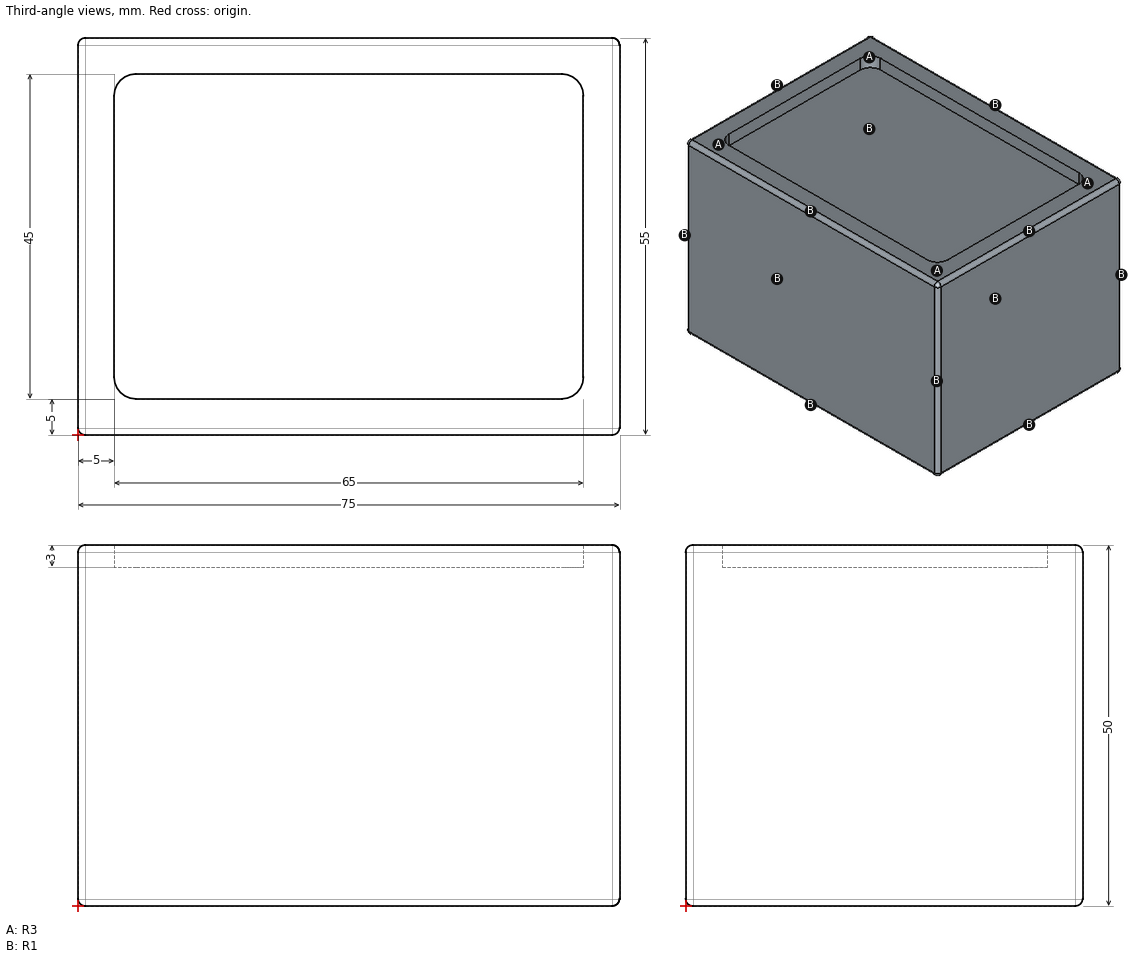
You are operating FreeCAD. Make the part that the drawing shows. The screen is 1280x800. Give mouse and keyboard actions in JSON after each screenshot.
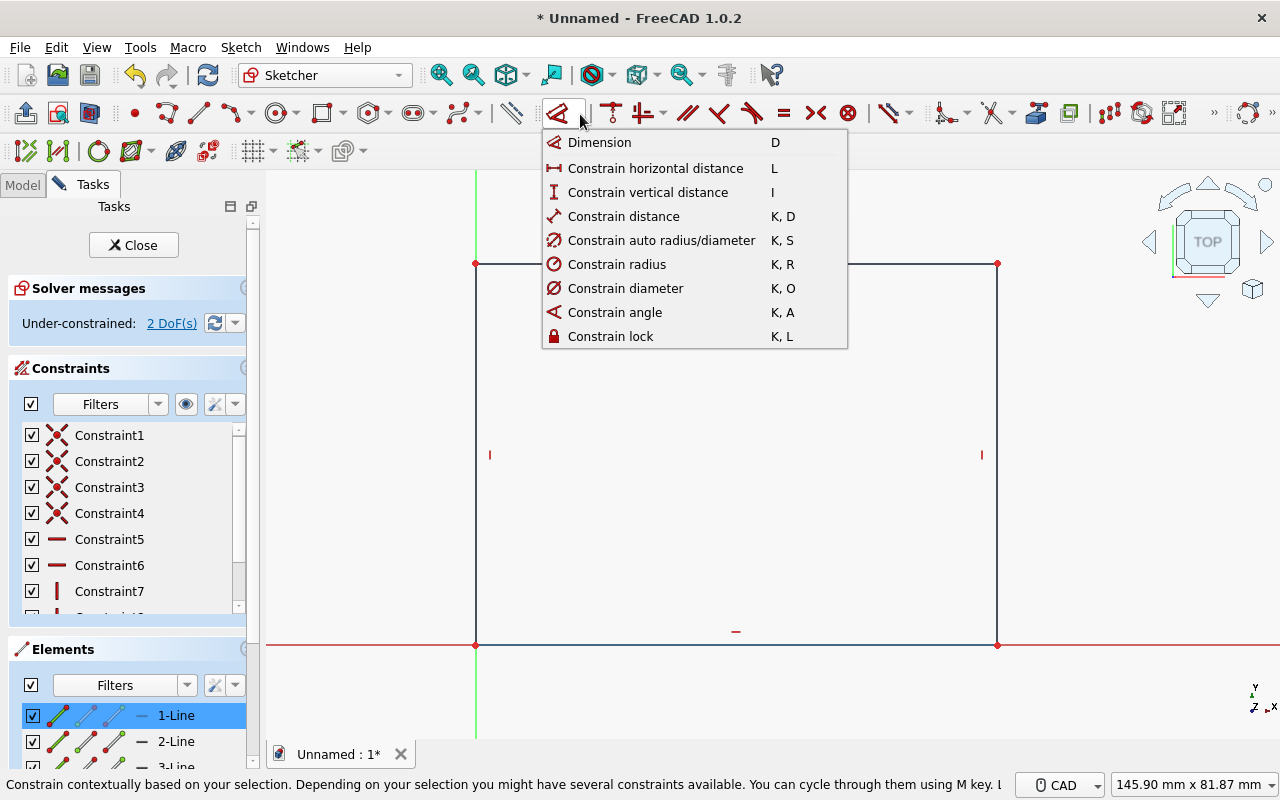
{"action": "left_click", "coordinate": [695, 168]}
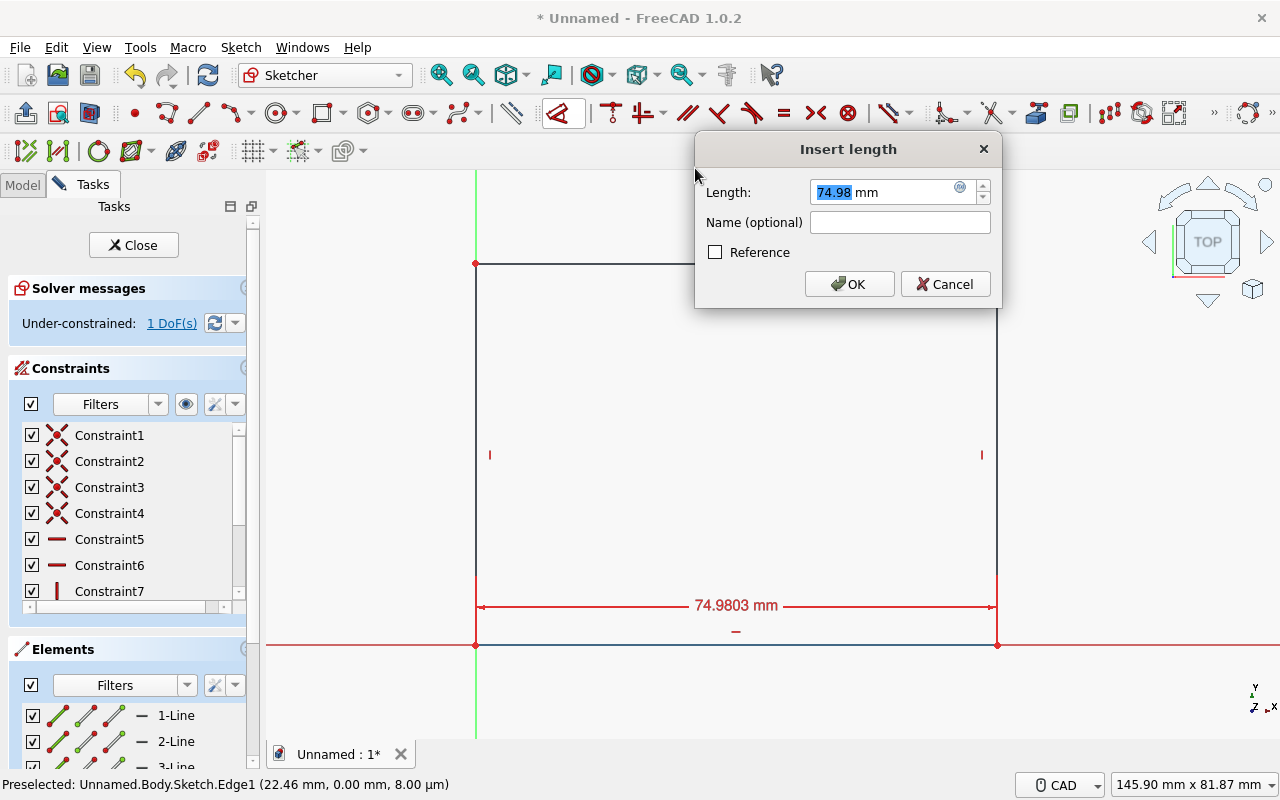
{"action": "type", "text": "75"}
{"action": "key", "text": "Return"}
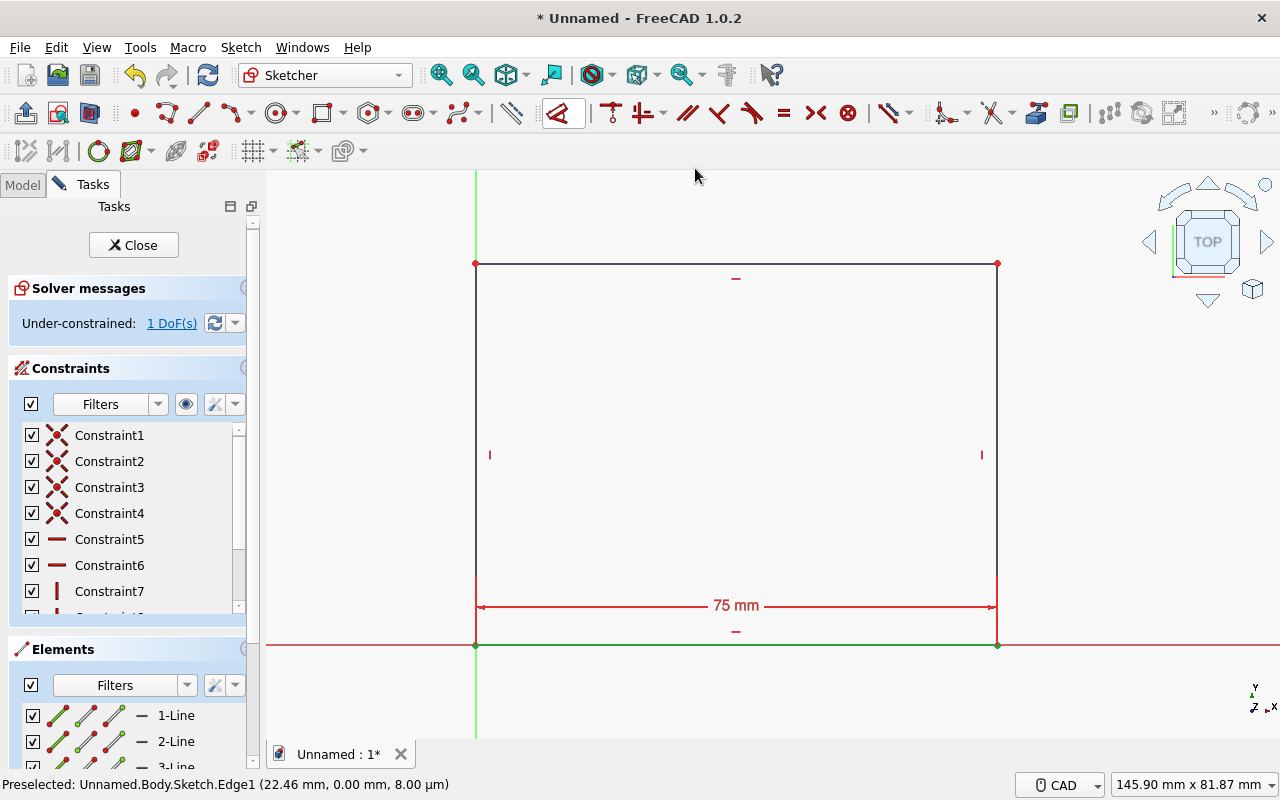
{"action": "left_click", "coordinate": [997, 531]}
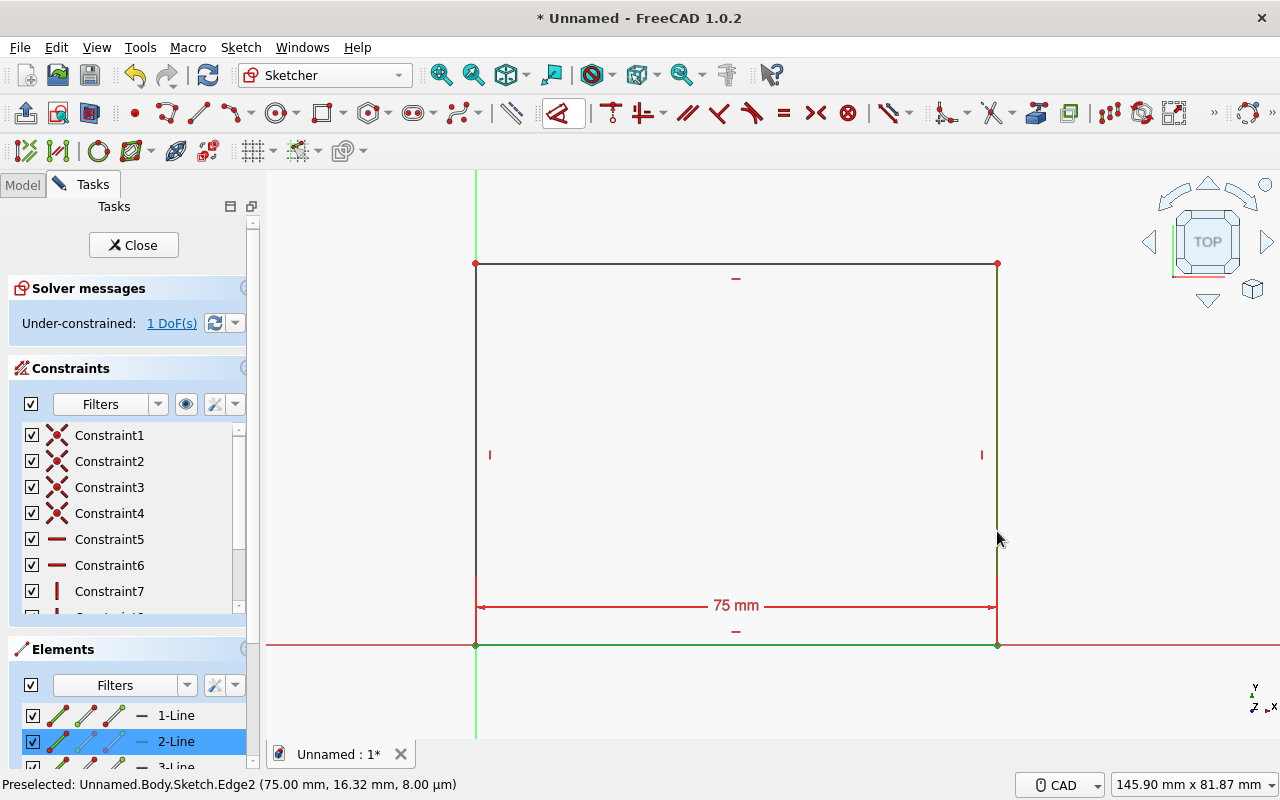
{"action": "left_click", "coordinate": [580, 114]}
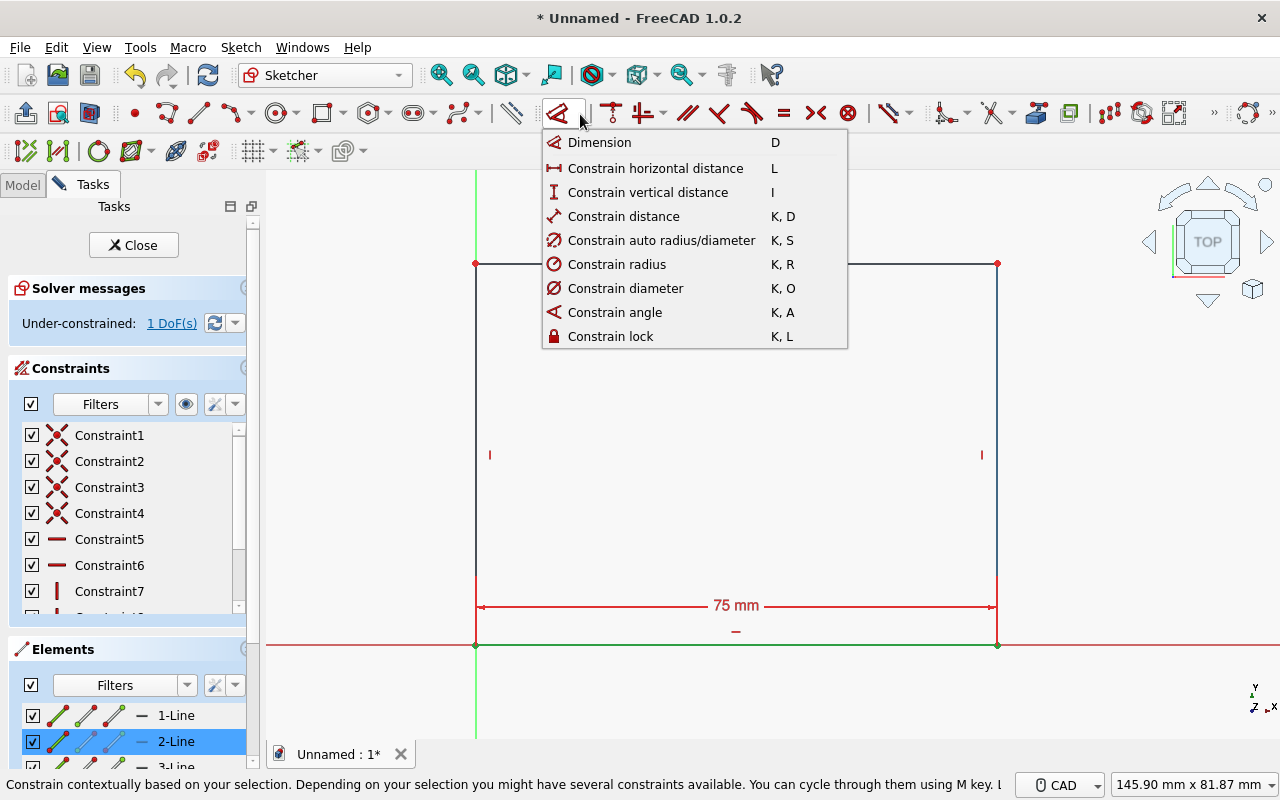
{"action": "left_click", "coordinate": [695, 192]}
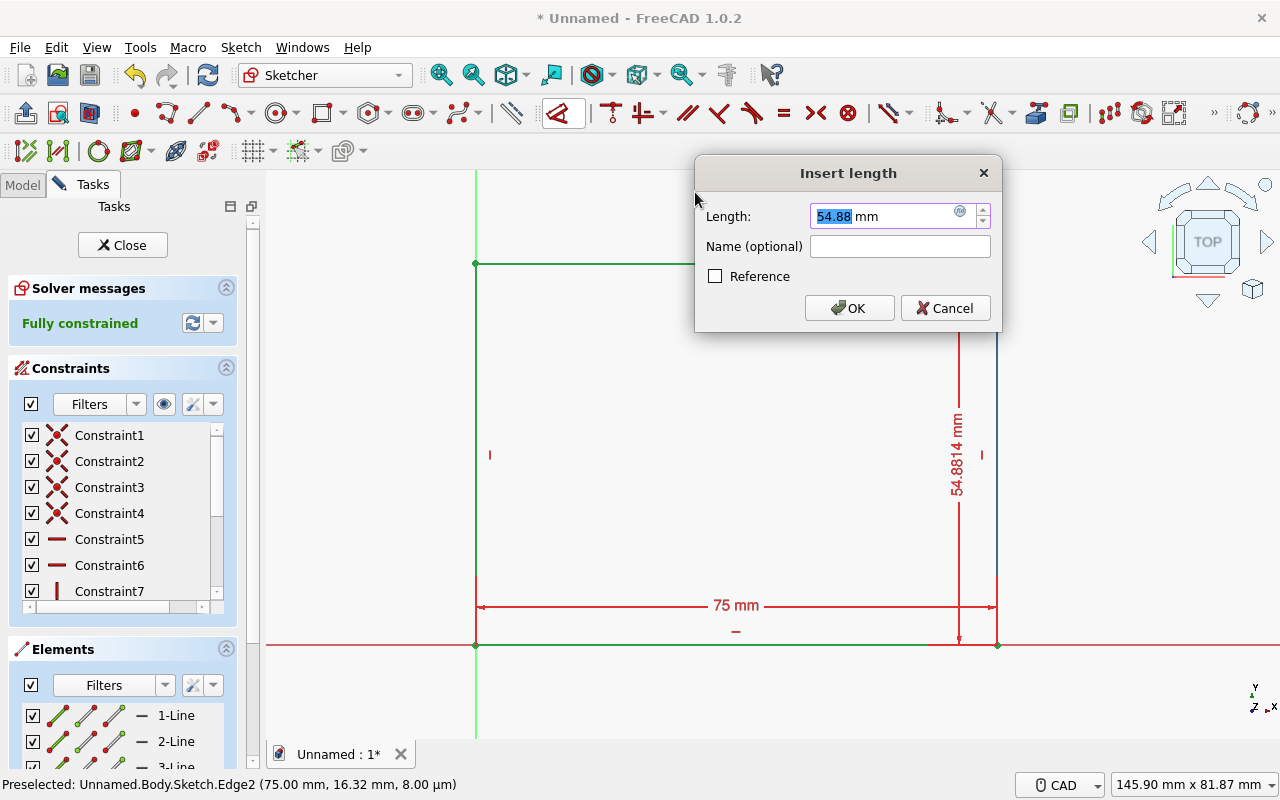
{"action": "type", "text": "55"}
{"action": "key", "text": "Return"}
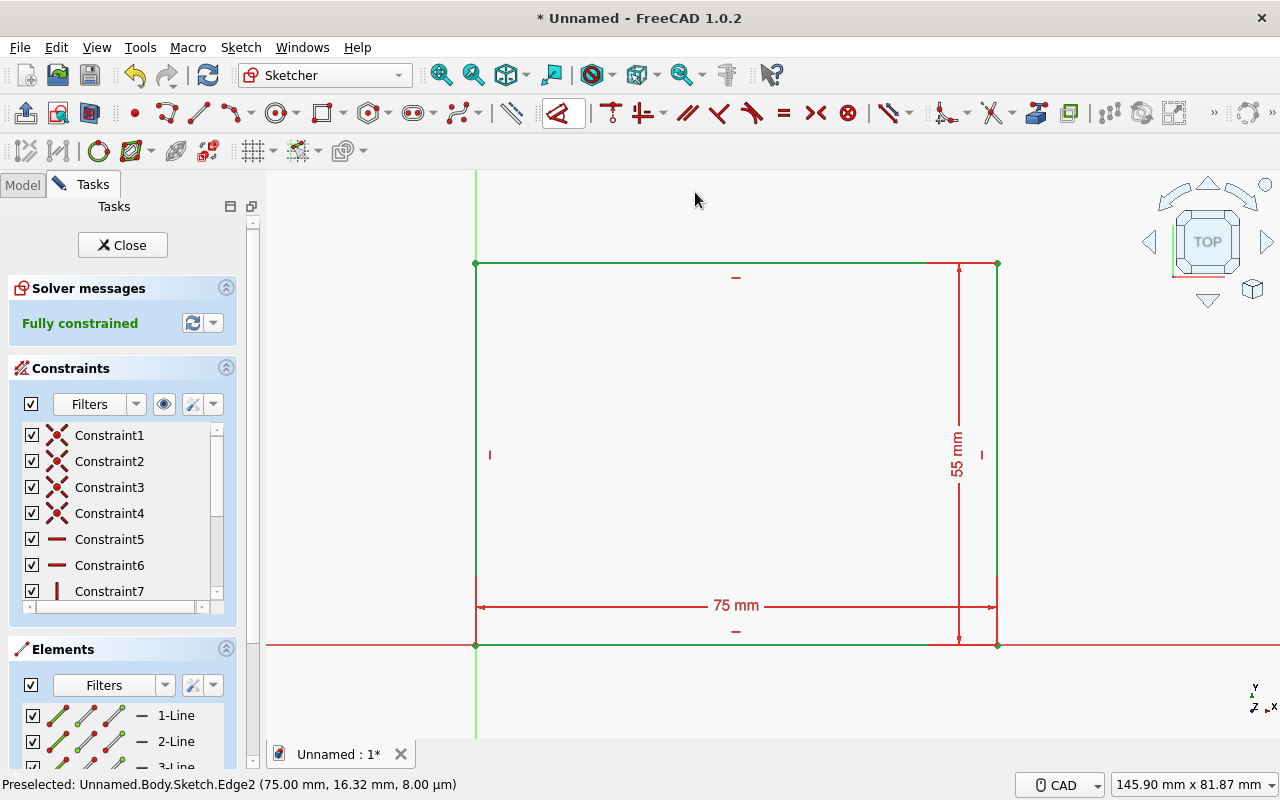
{"action": "left_click", "coordinate": [123, 245]}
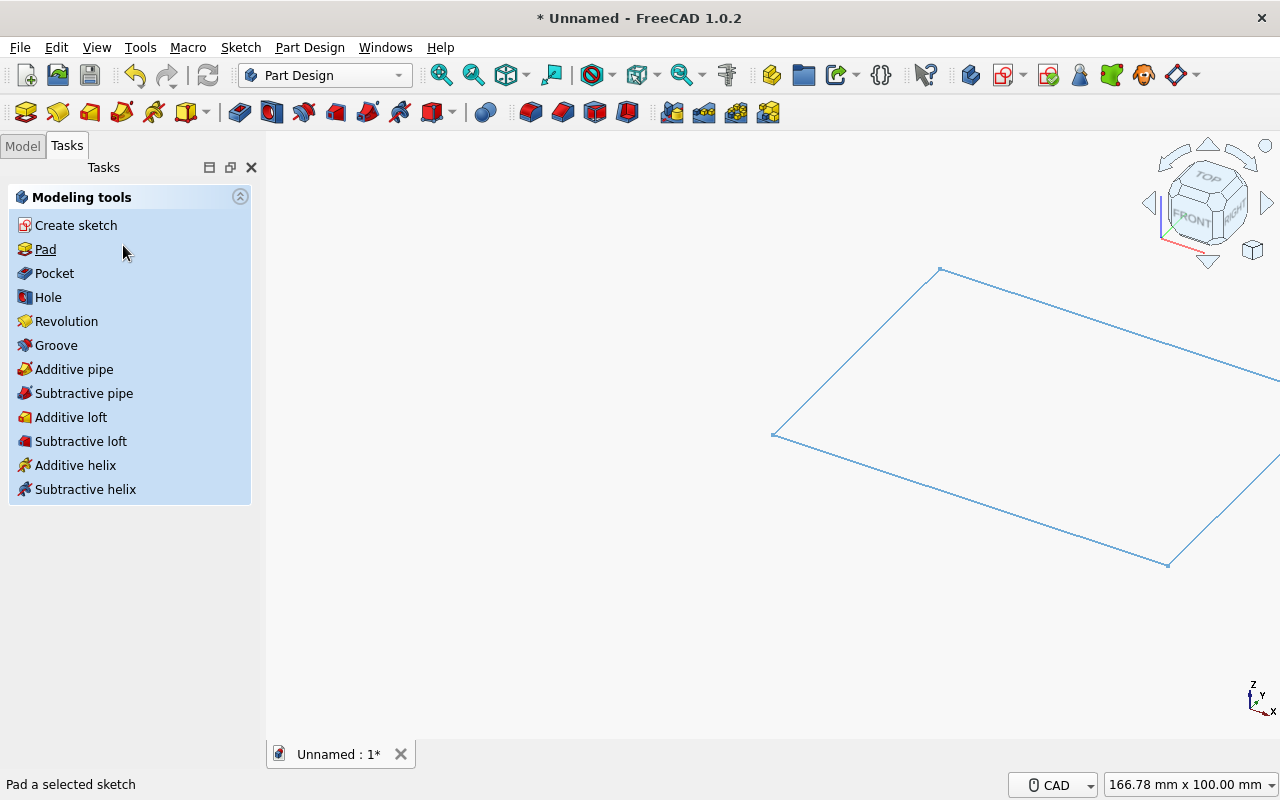
{"action": "left_click", "coordinate": [26, 112]}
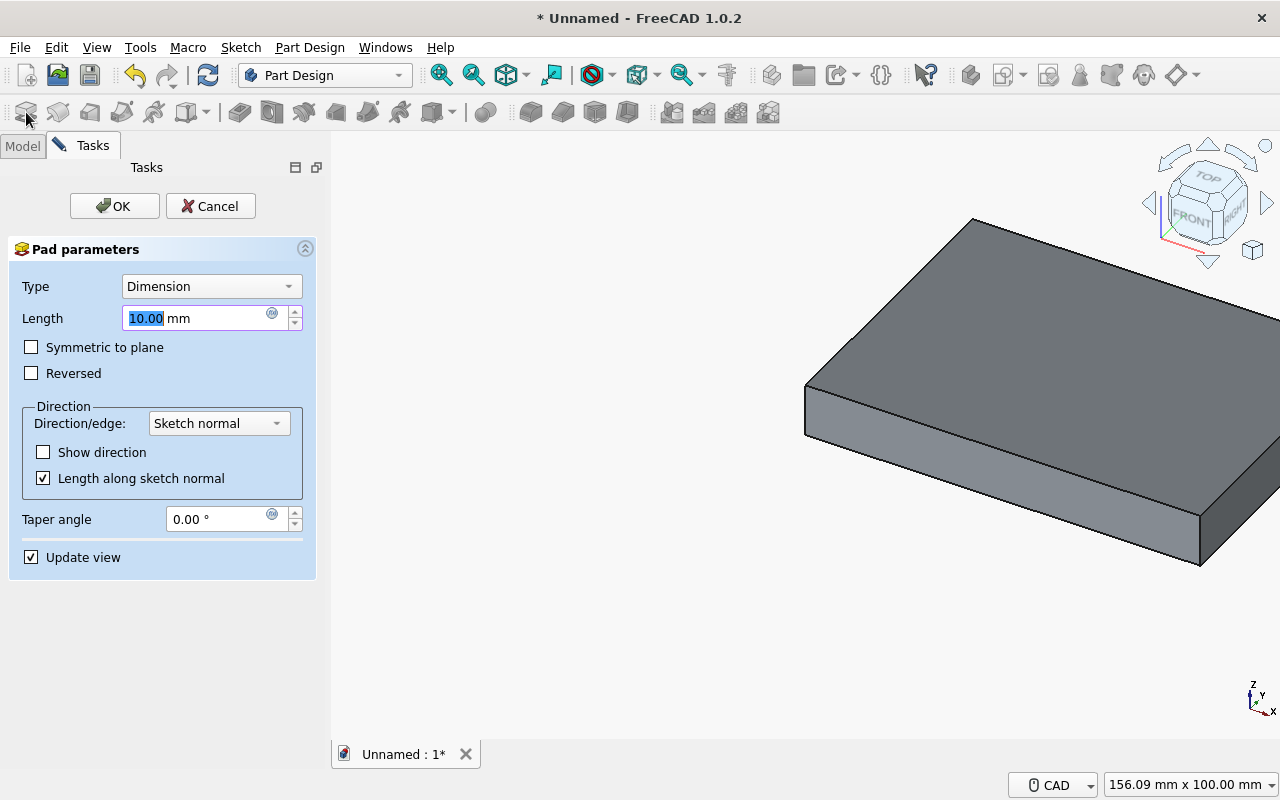
{"action": "type", "text": "50"}
{"action": "key", "text": "Tab"}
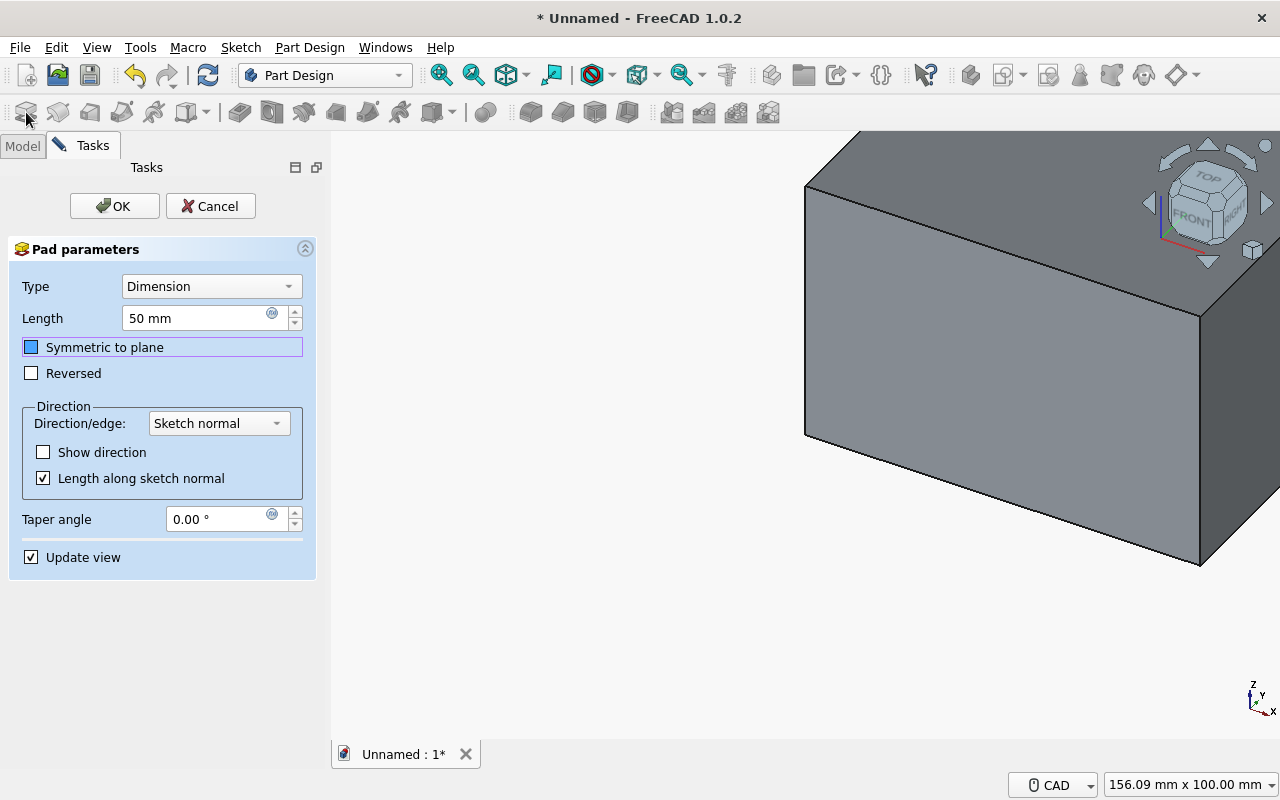
{"action": "left_click", "coordinate": [115, 206]}